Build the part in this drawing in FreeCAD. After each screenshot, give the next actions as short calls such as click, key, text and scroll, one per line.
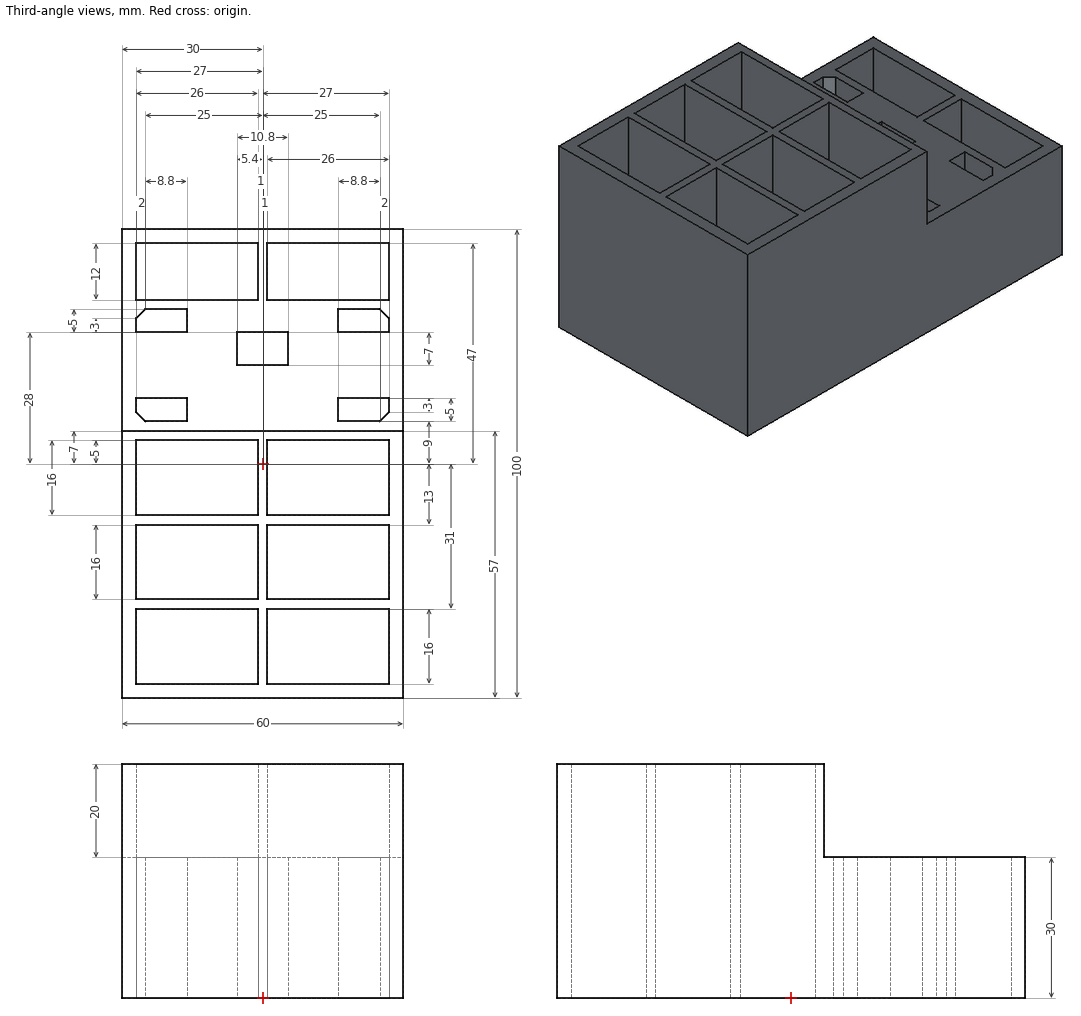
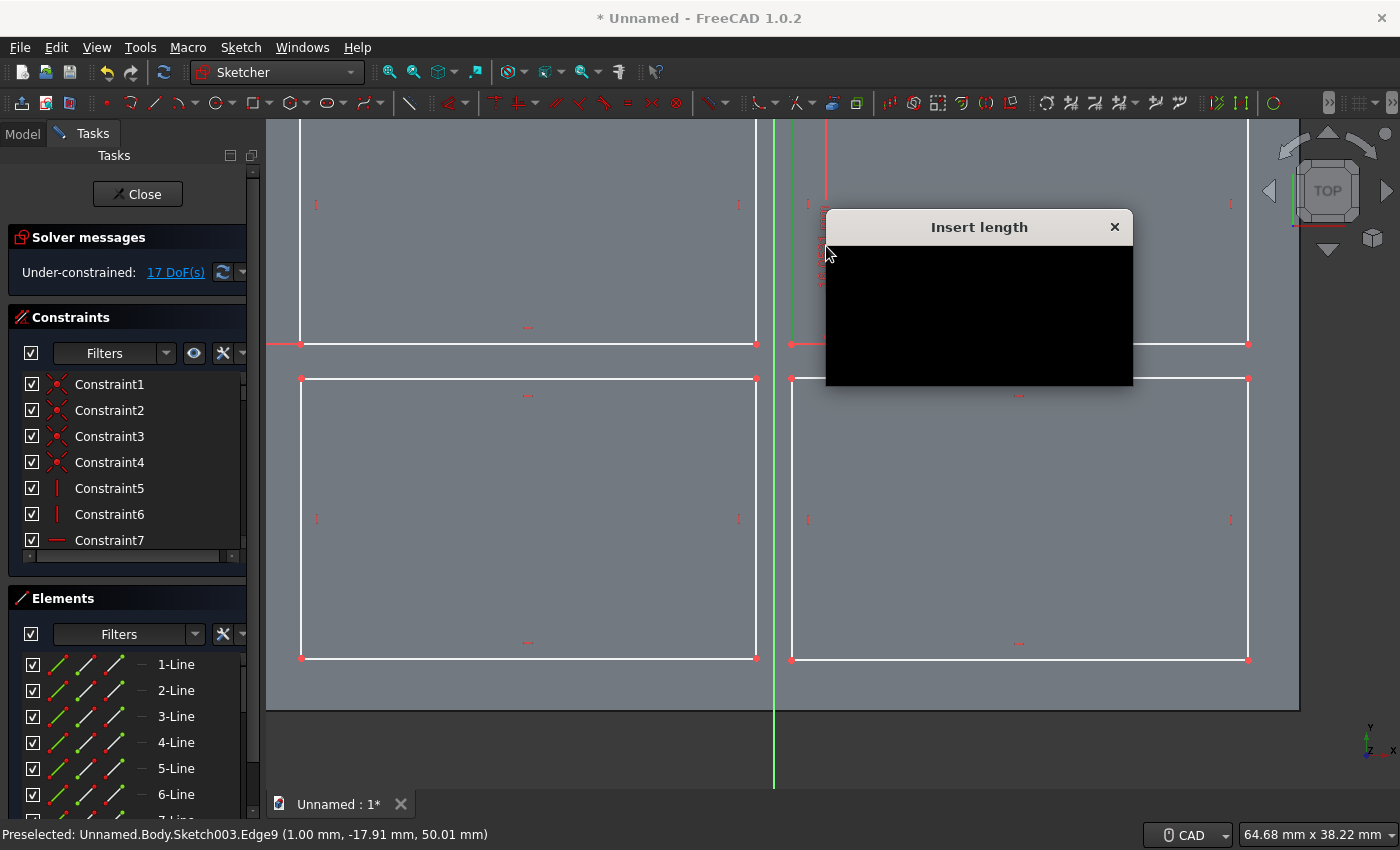
text(16)
key(Return)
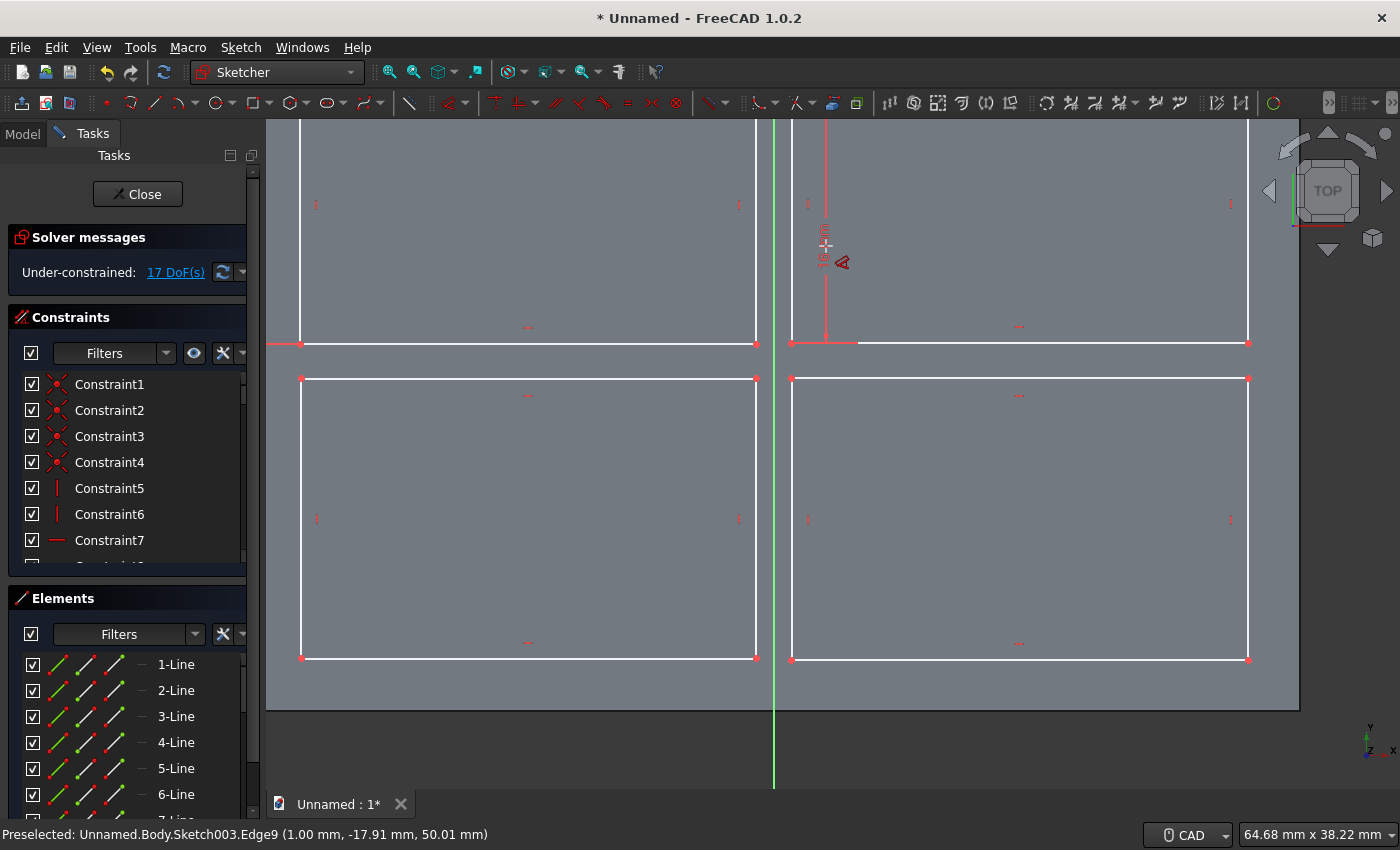
click(929, 343)
click(1013, 309)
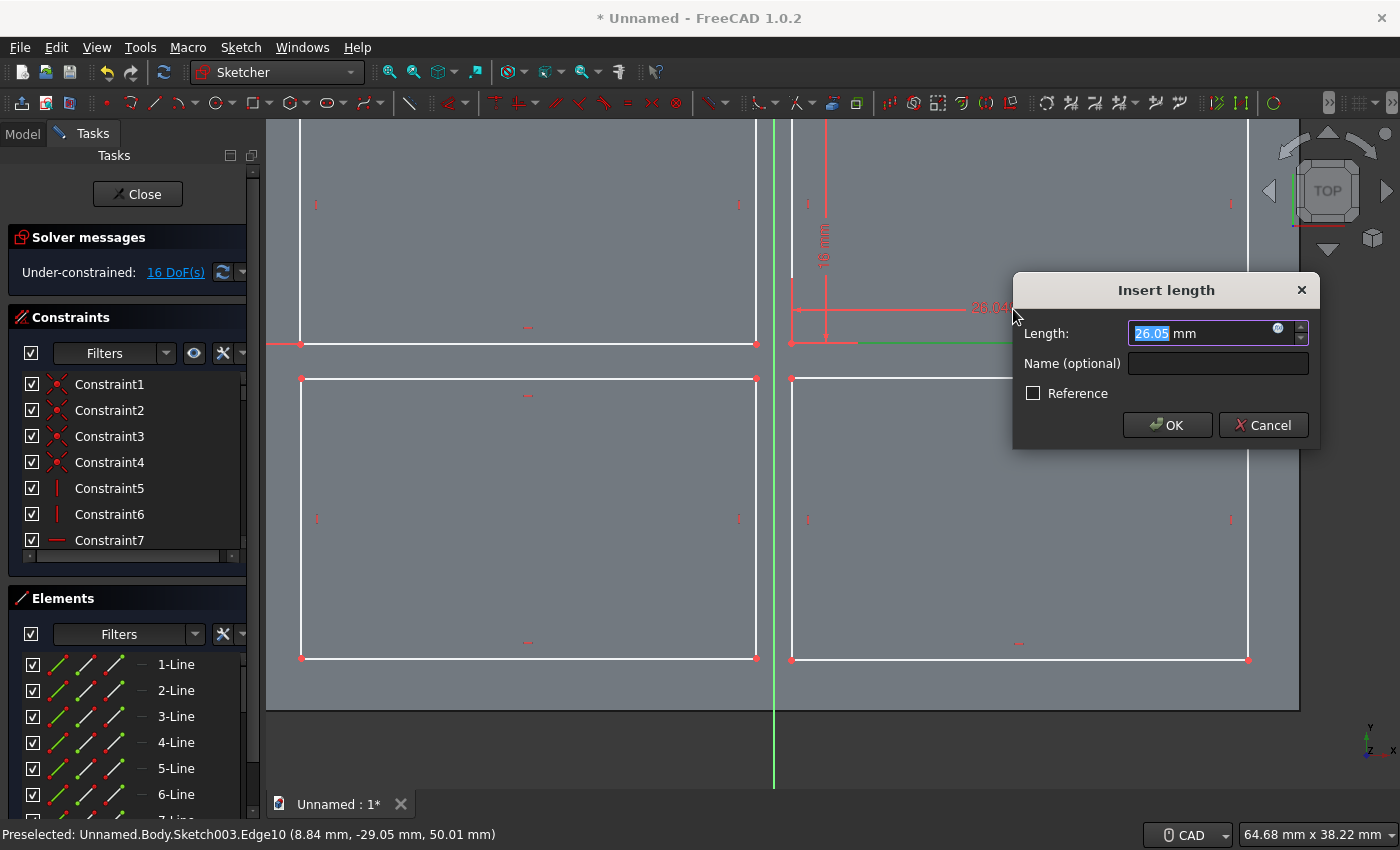
text(26)
key(Return)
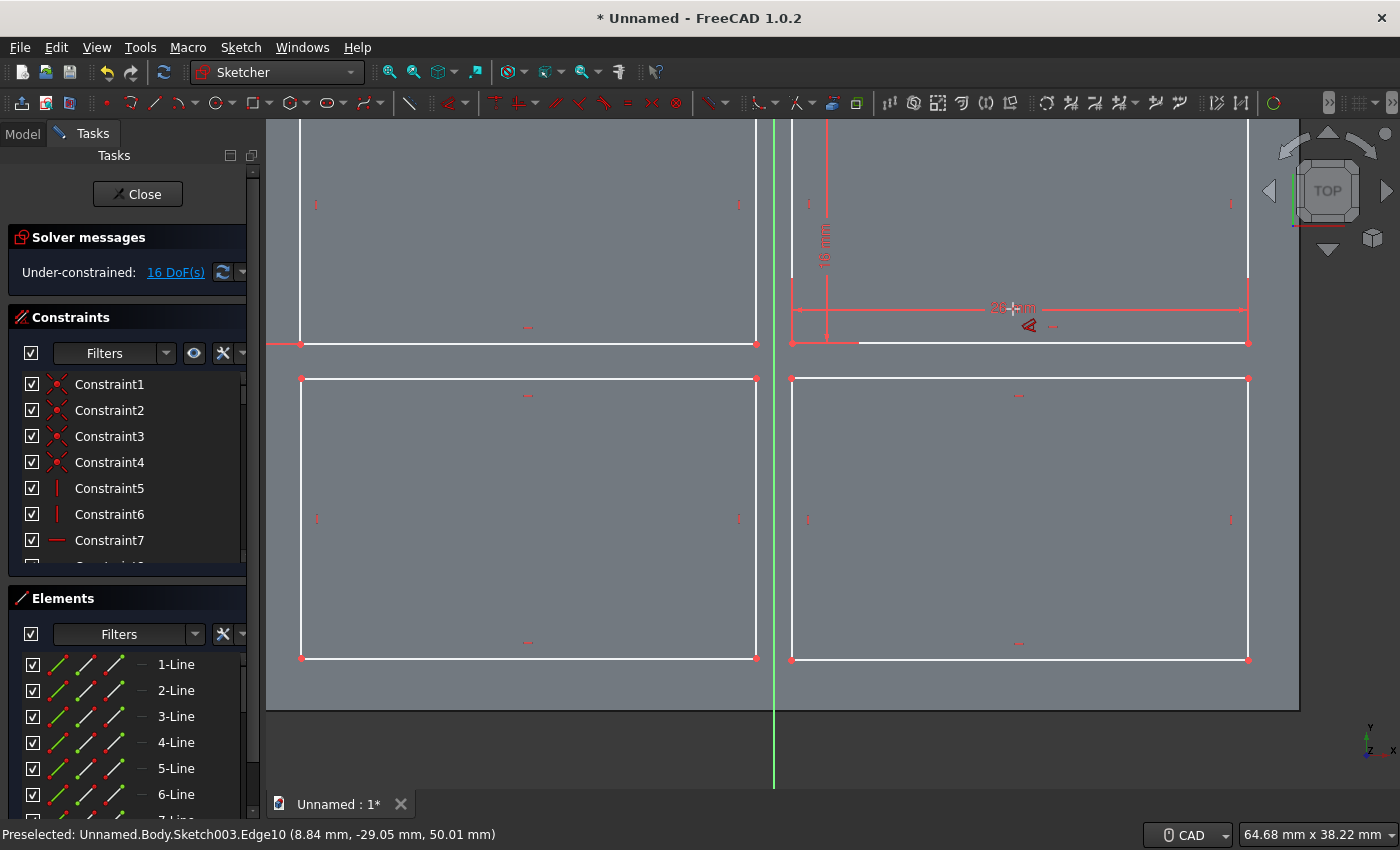
click(792, 463)
click(826, 519)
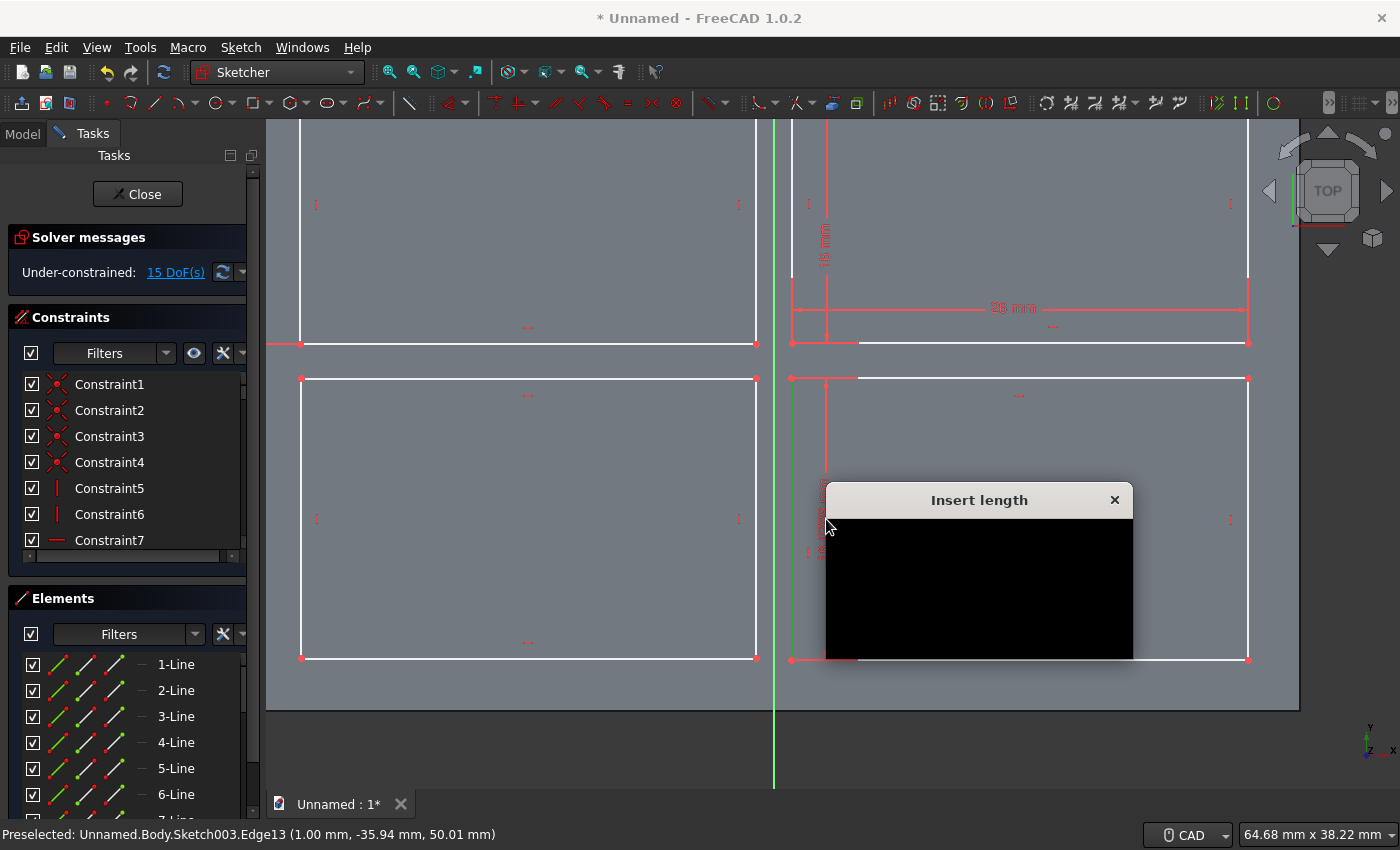
text(16)
key(Return)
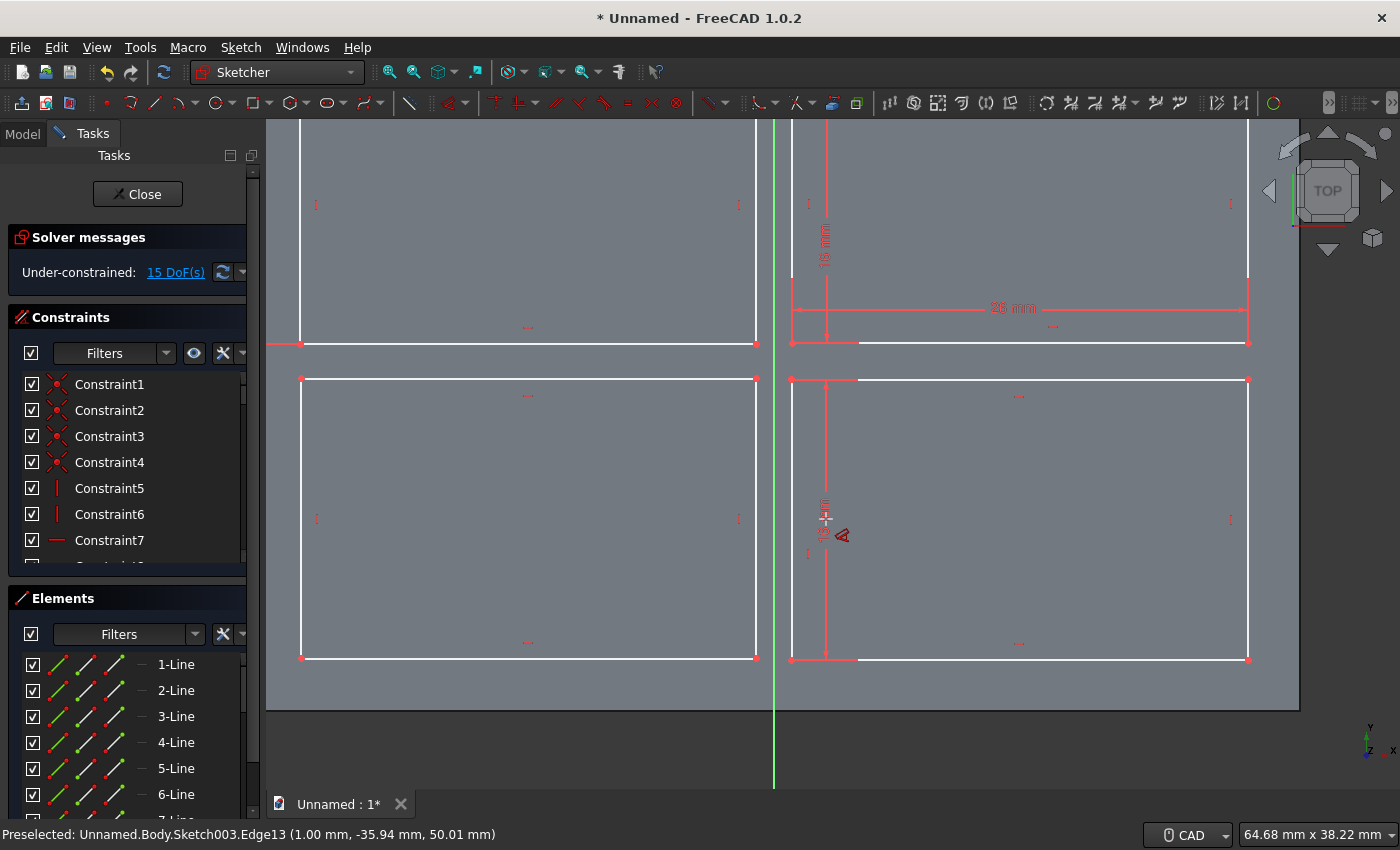
click(929, 660)
click(1013, 694)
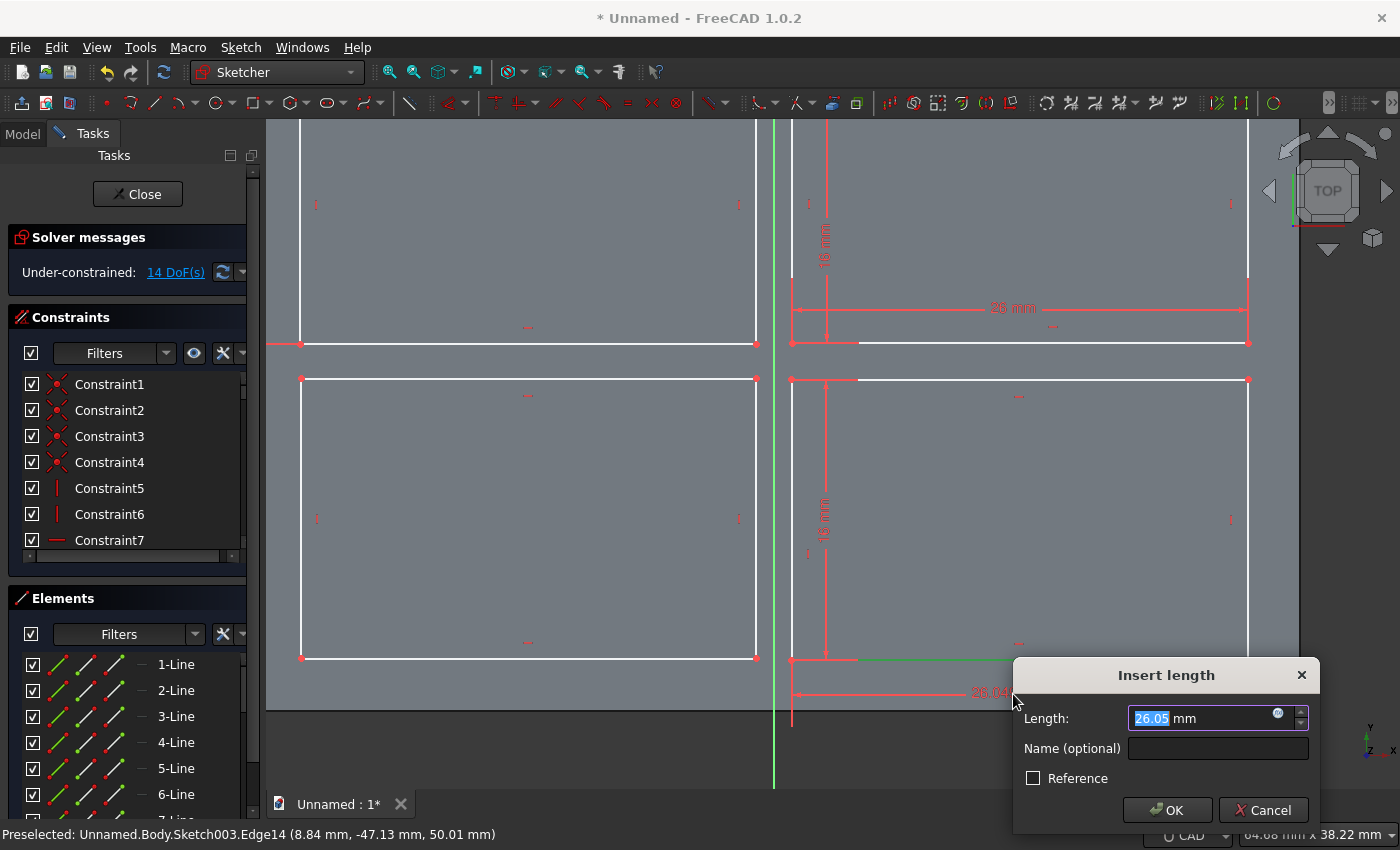
text(26)
key(Return)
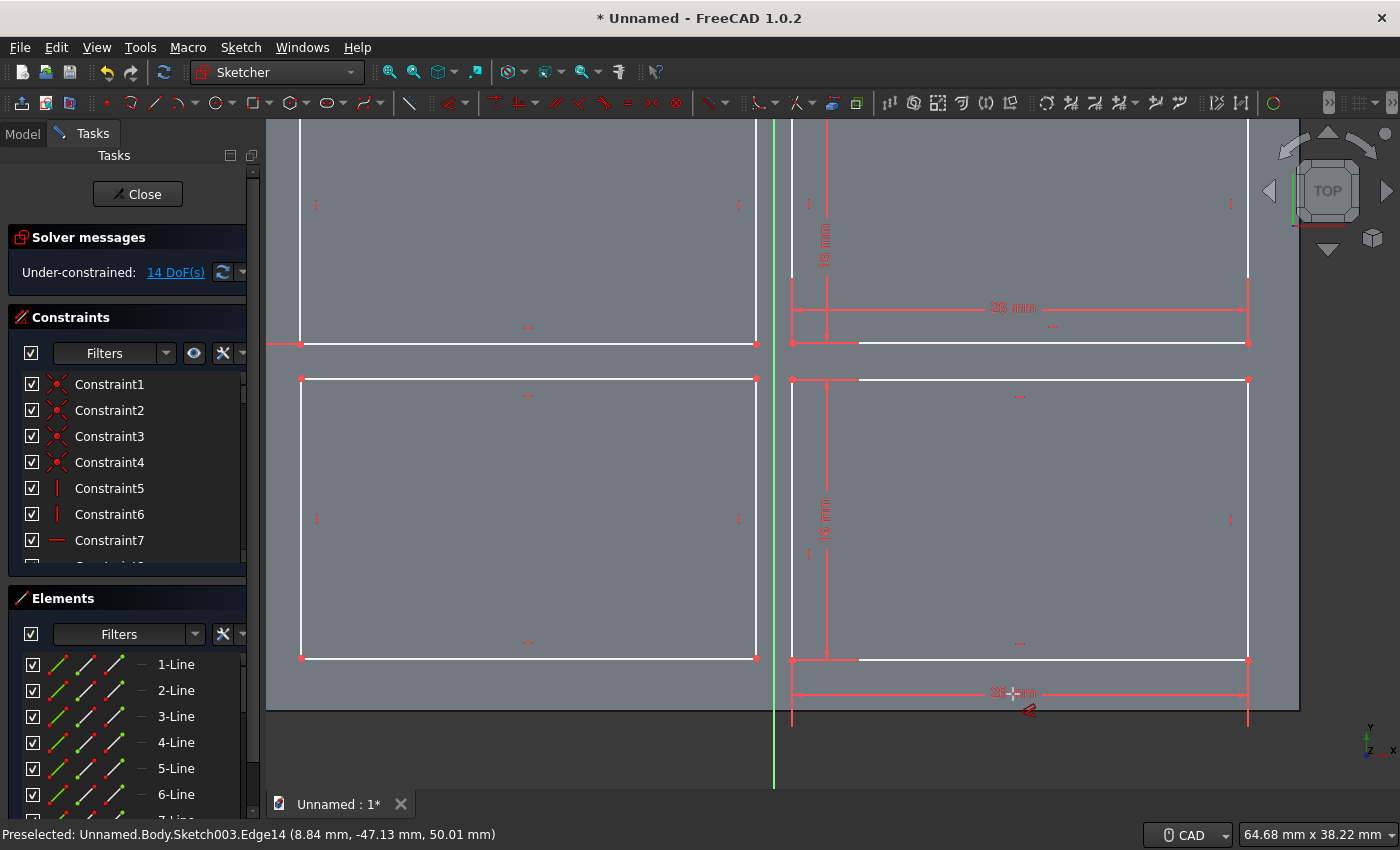
click(301, 463)
click(335, 519)